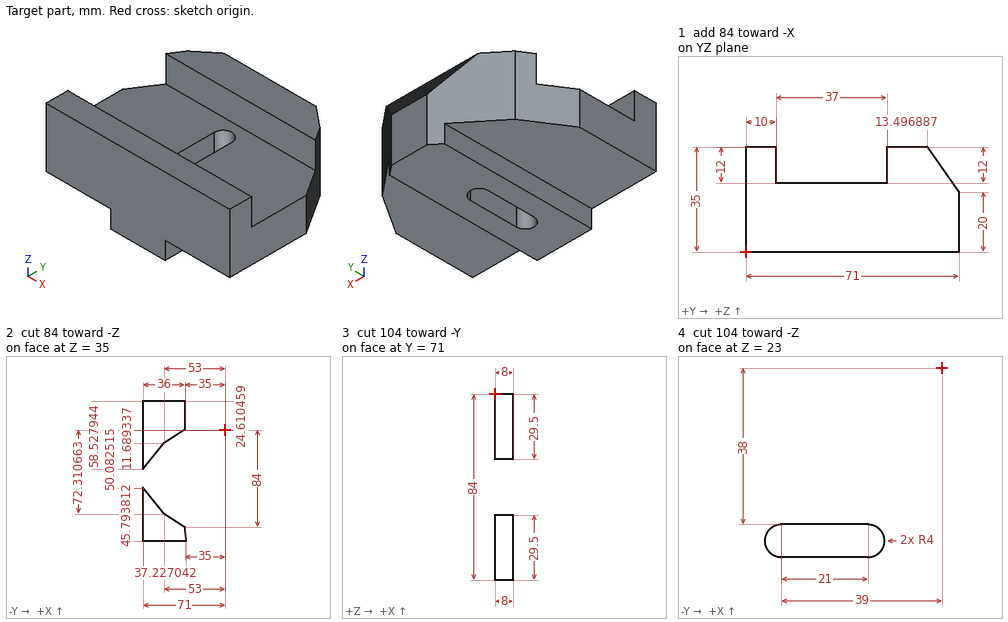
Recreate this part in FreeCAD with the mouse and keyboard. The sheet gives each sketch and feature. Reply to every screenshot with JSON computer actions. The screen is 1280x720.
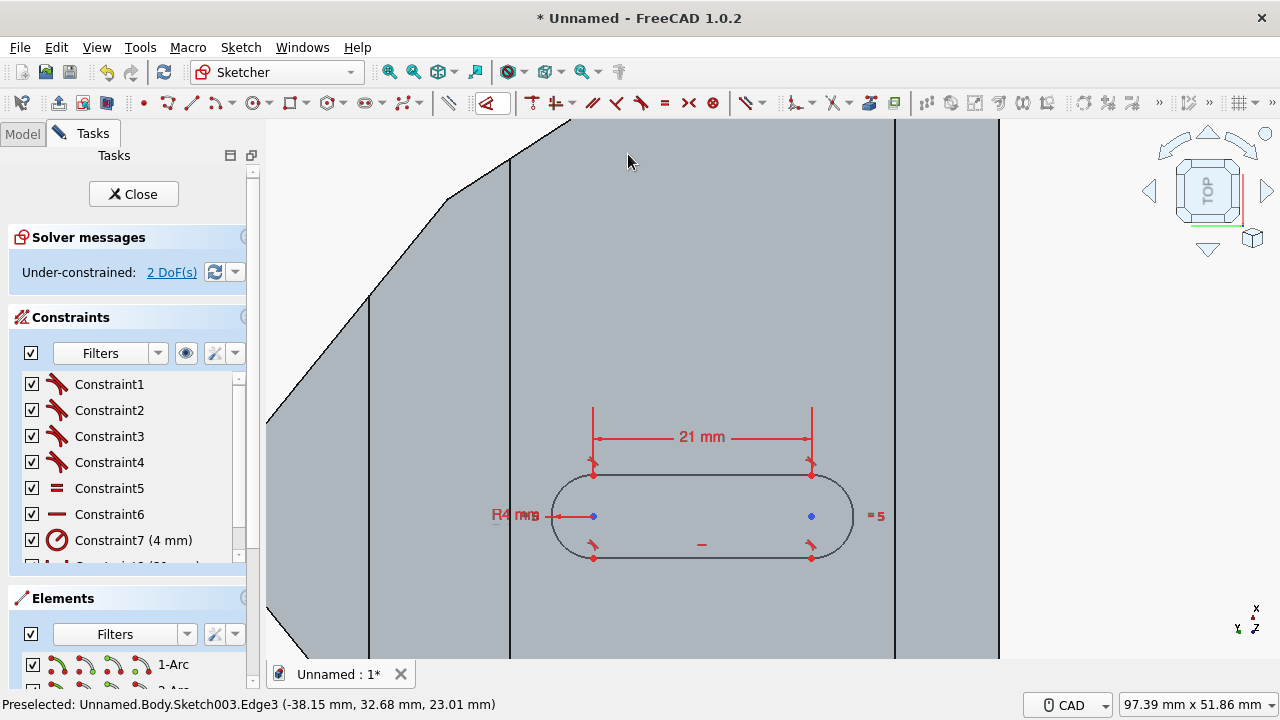
{"action": "left_click", "coordinate": [593, 475]}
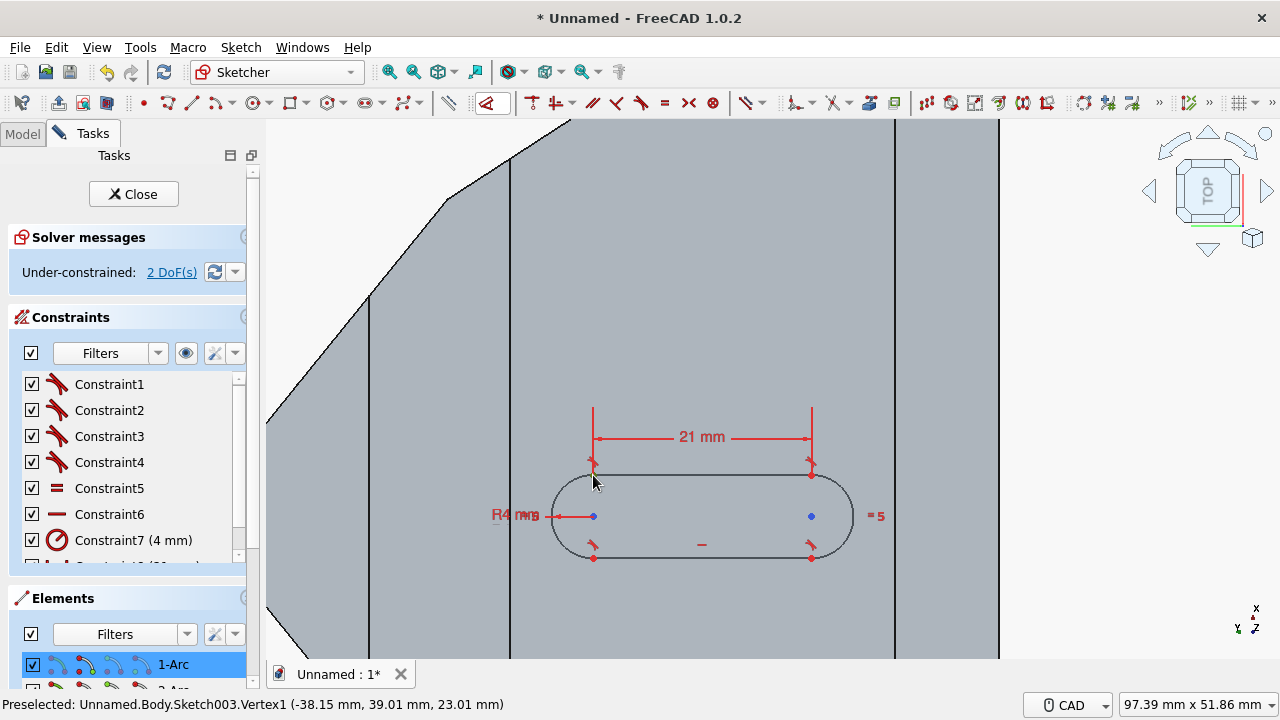
{"action": "left_click", "coordinate": [504, 104]}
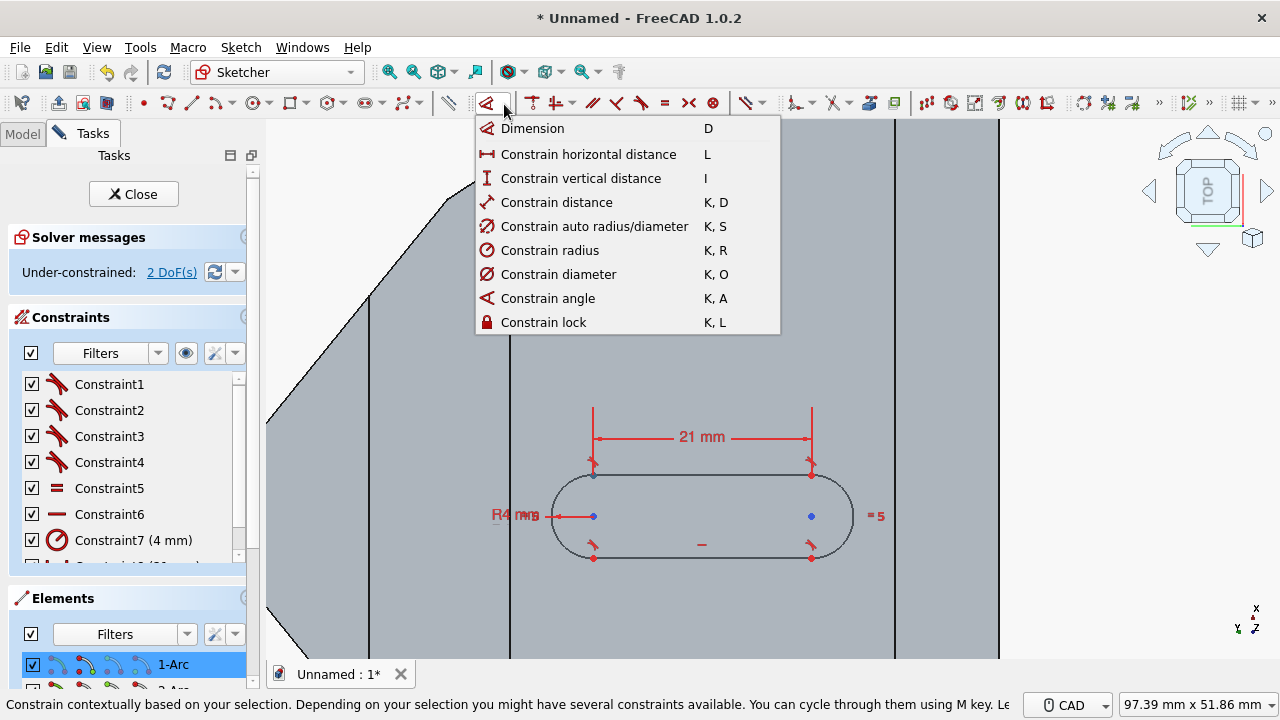
{"action": "left_click", "coordinate": [628, 154]}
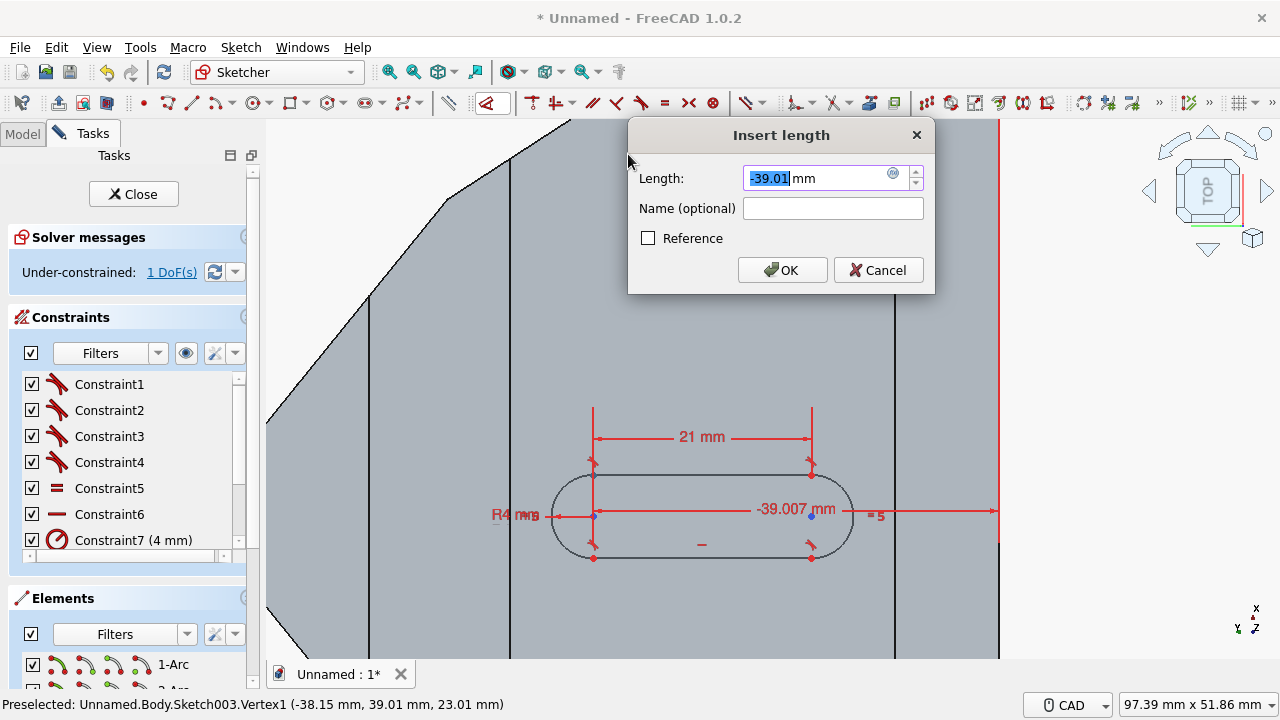
{"action": "type", "text": "-39"}
{"action": "key", "text": "Return"}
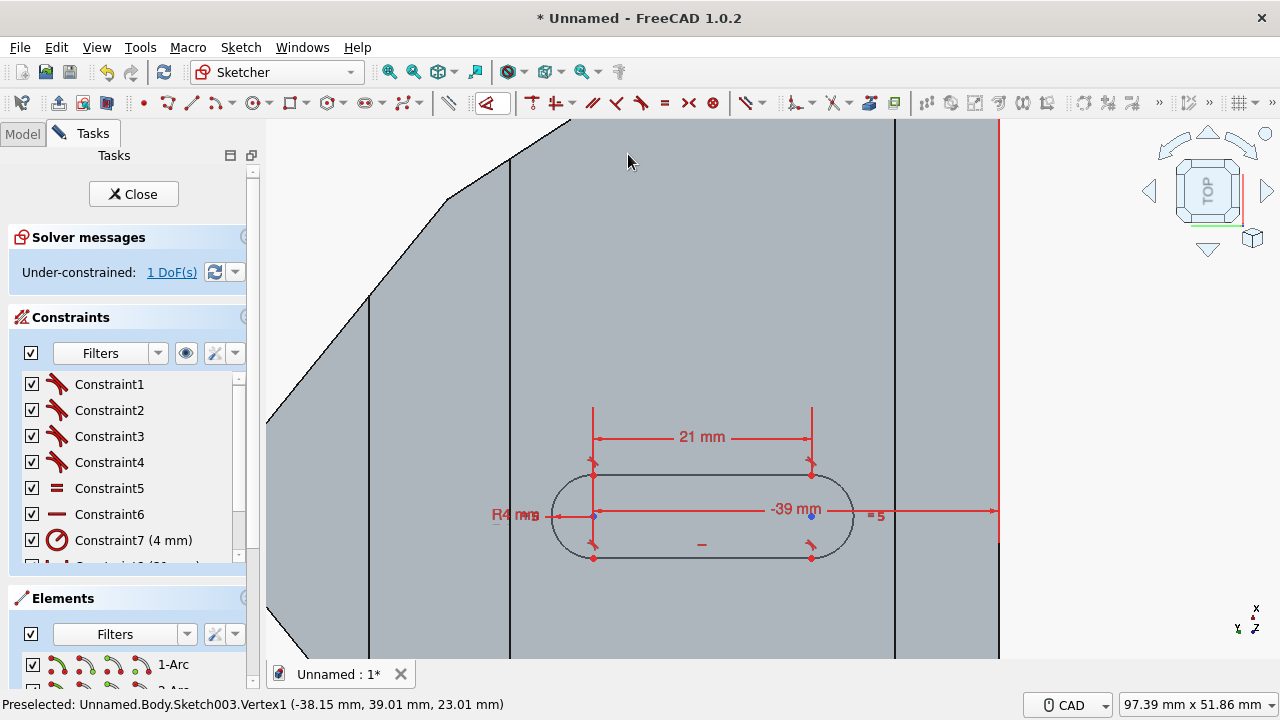
{"action": "left_click", "coordinate": [593, 475]}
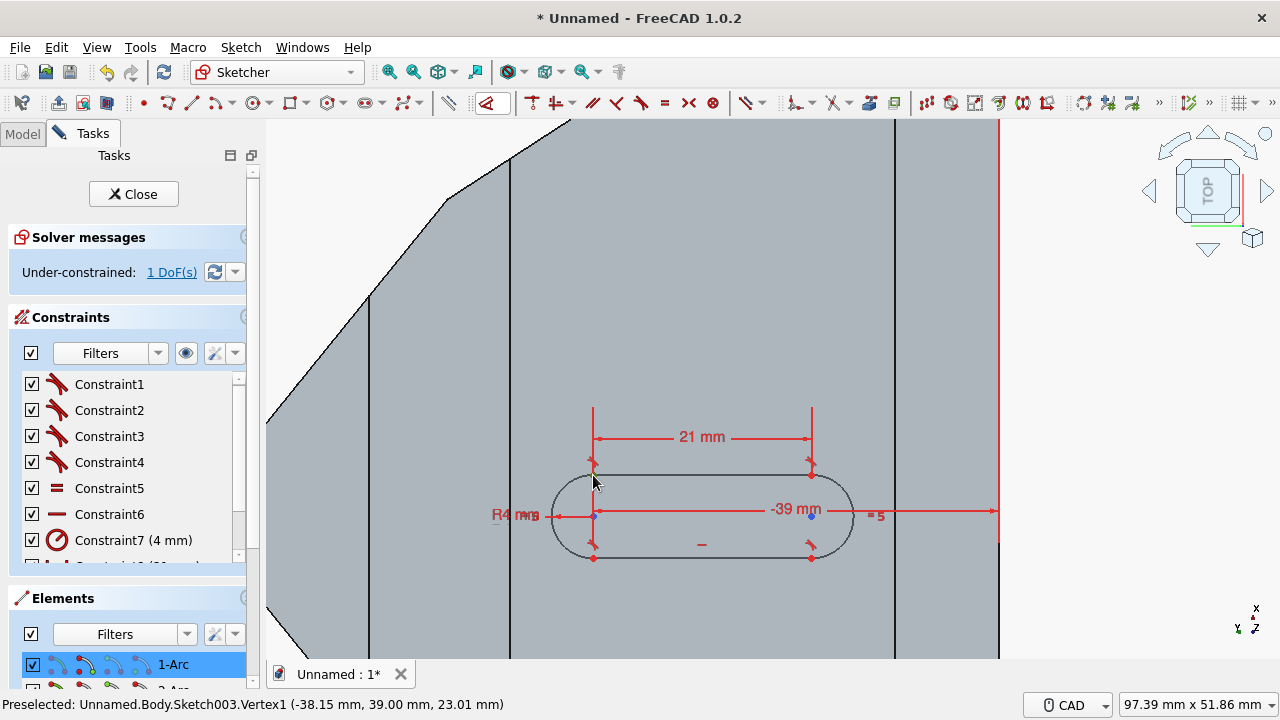
{"action": "key", "text": "i"}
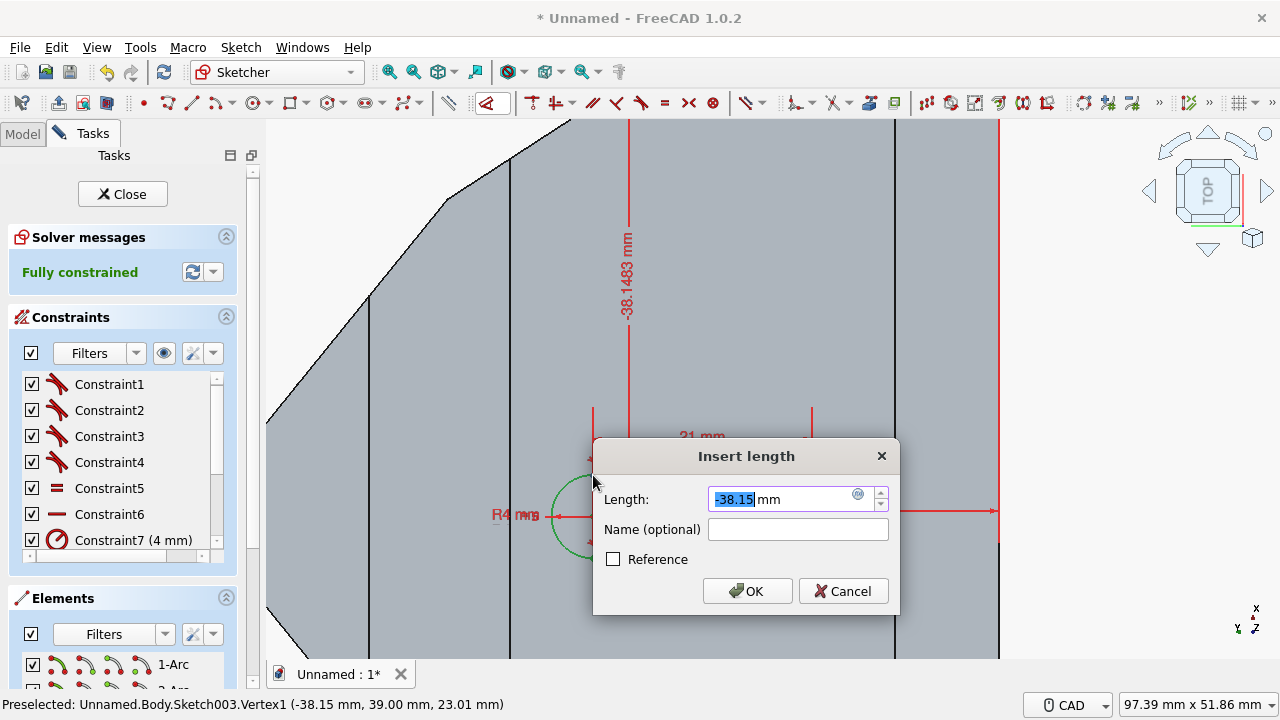
{"action": "type", "text": "-38"}
{"action": "key", "text": "Return"}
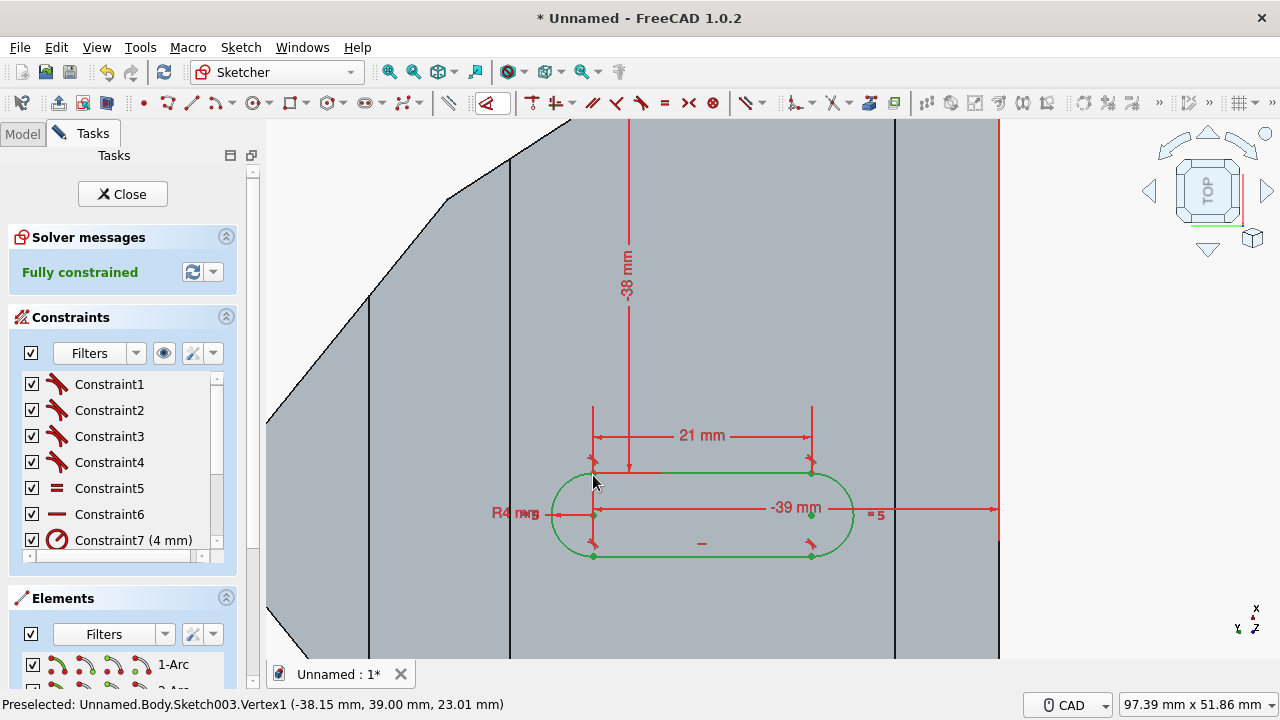
{"action": "left_click", "coordinate": [123, 194]}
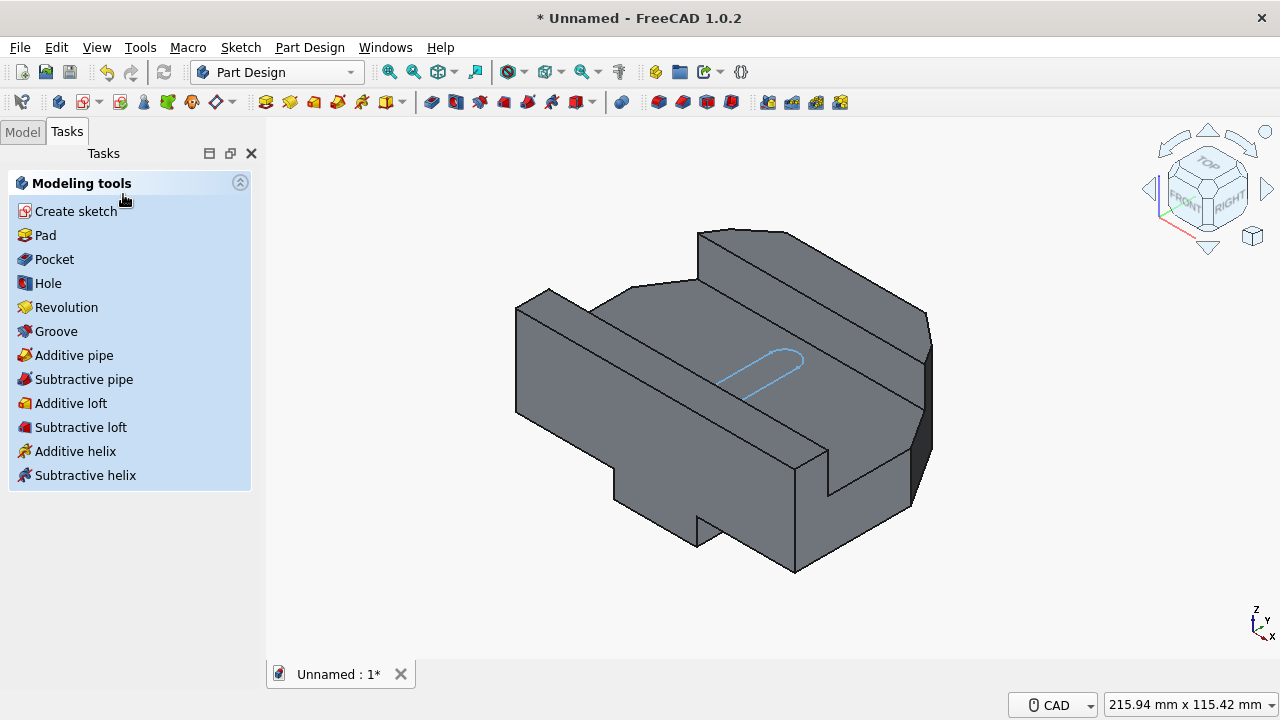
{"action": "left_click", "coordinate": [432, 102]}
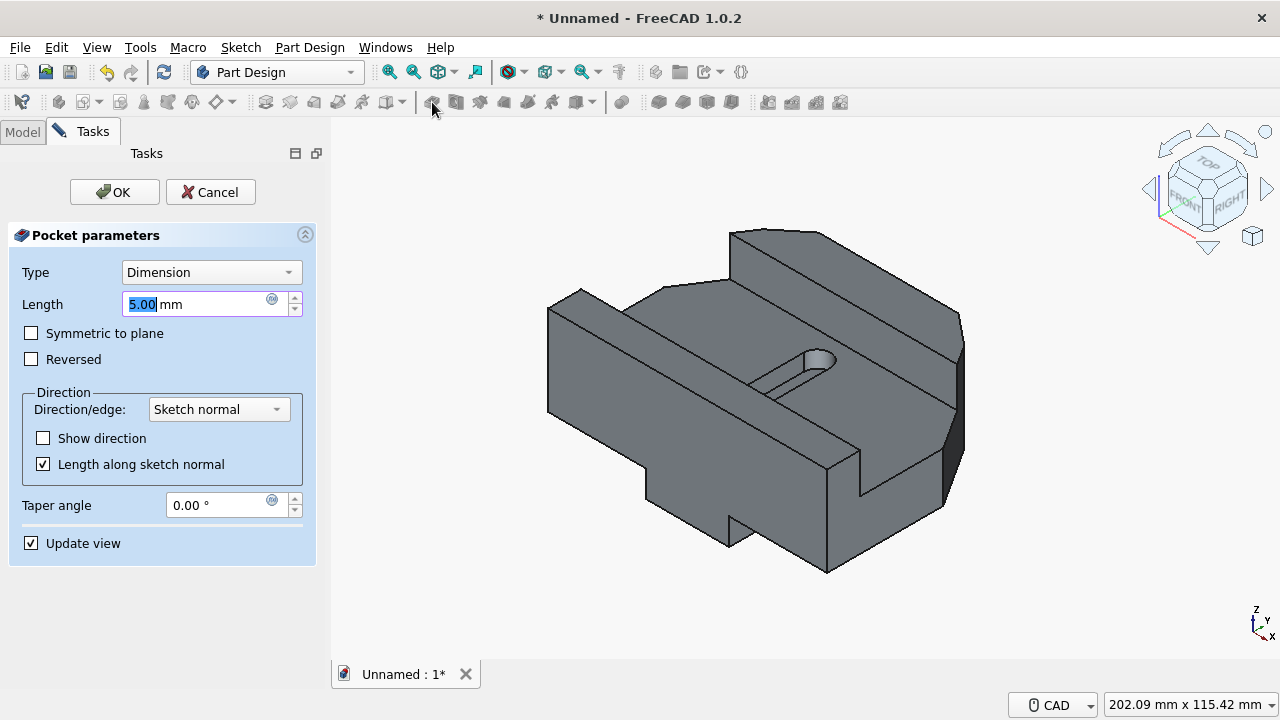
{"action": "type", "text": "104"}
{"action": "key", "text": "Tab"}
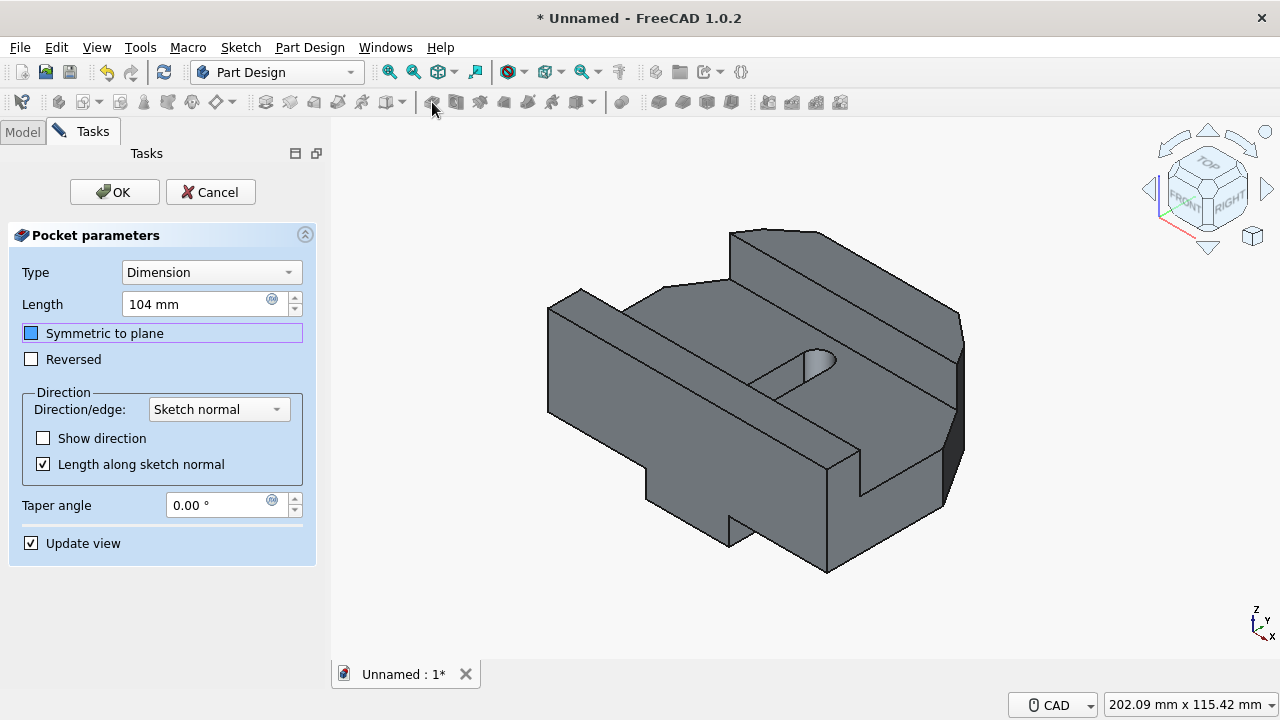
{"action": "left_click", "coordinate": [115, 192]}